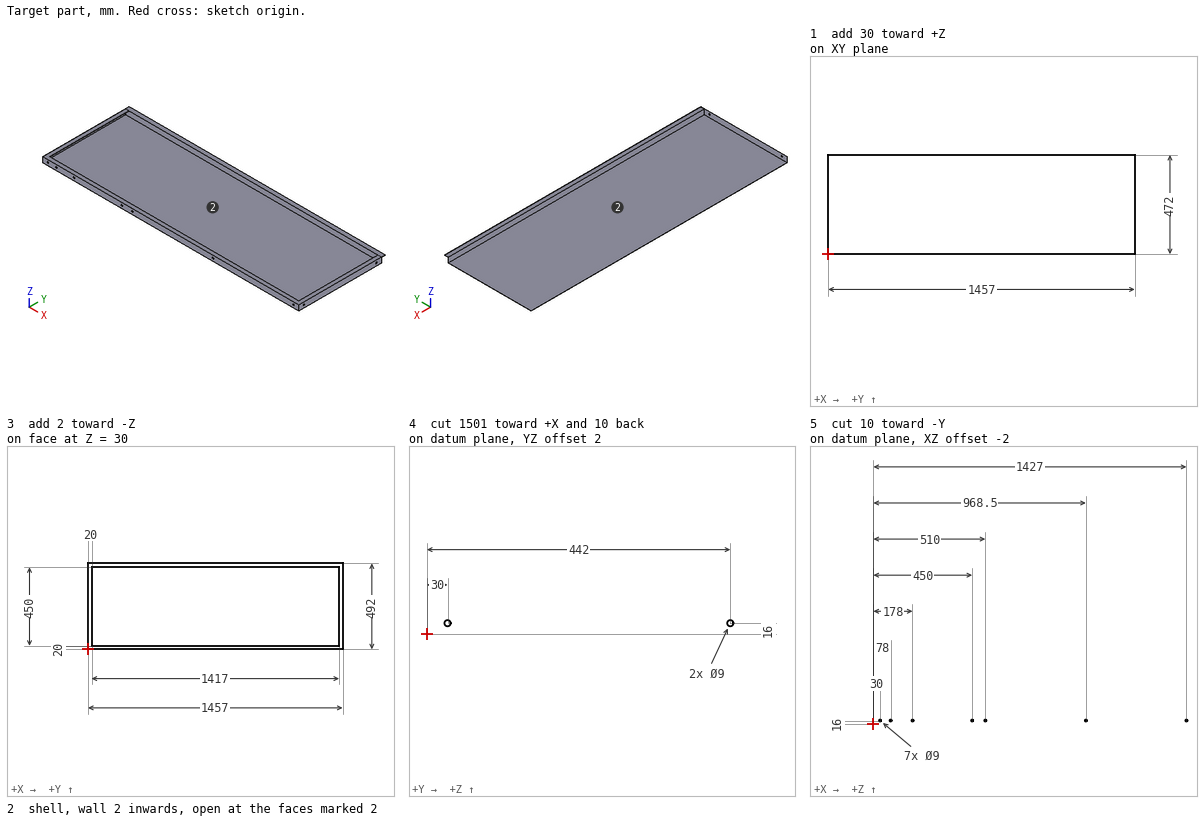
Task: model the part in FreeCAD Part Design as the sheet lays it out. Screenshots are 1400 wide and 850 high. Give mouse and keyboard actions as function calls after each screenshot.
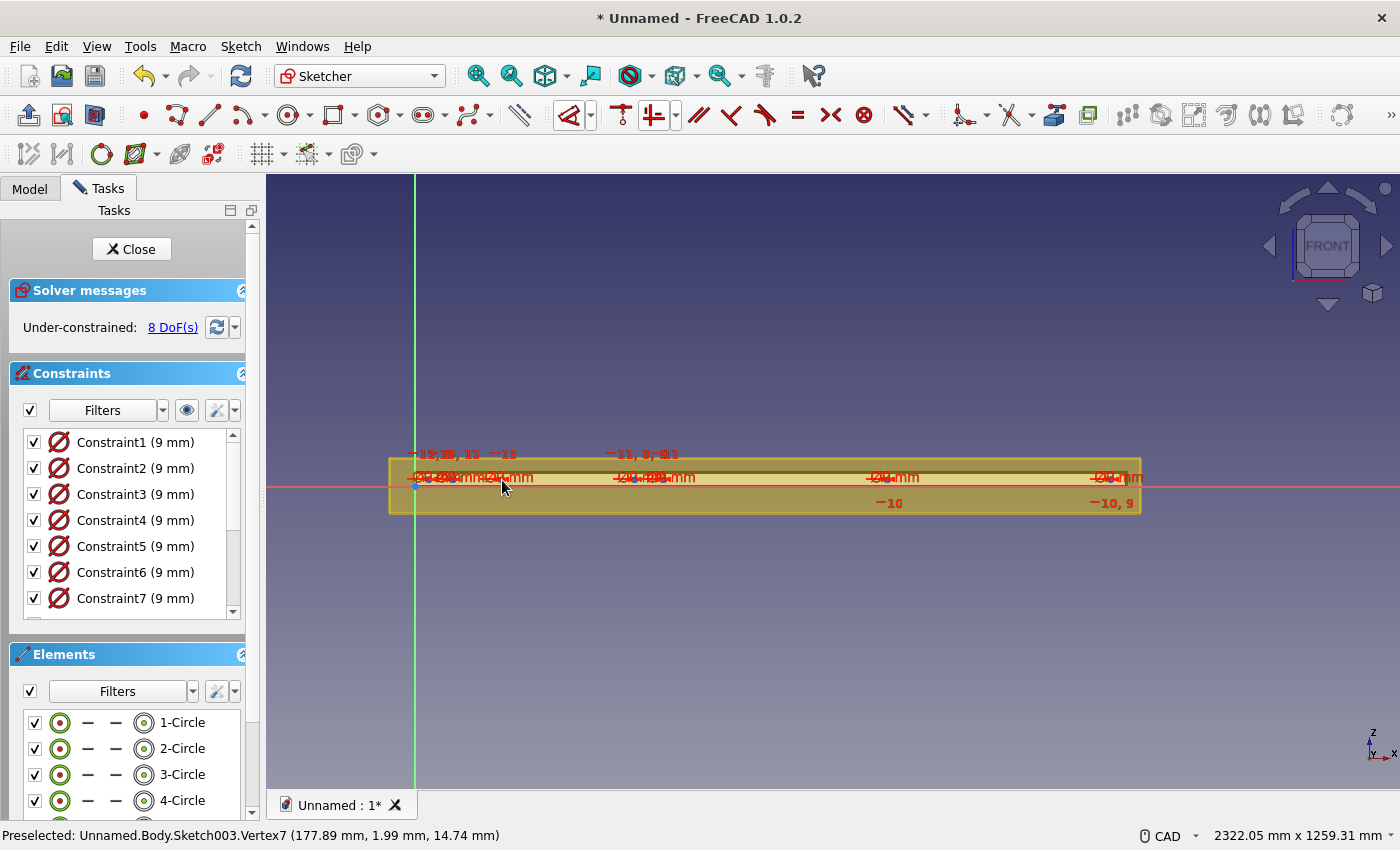
scroll(430, 479, up, 5)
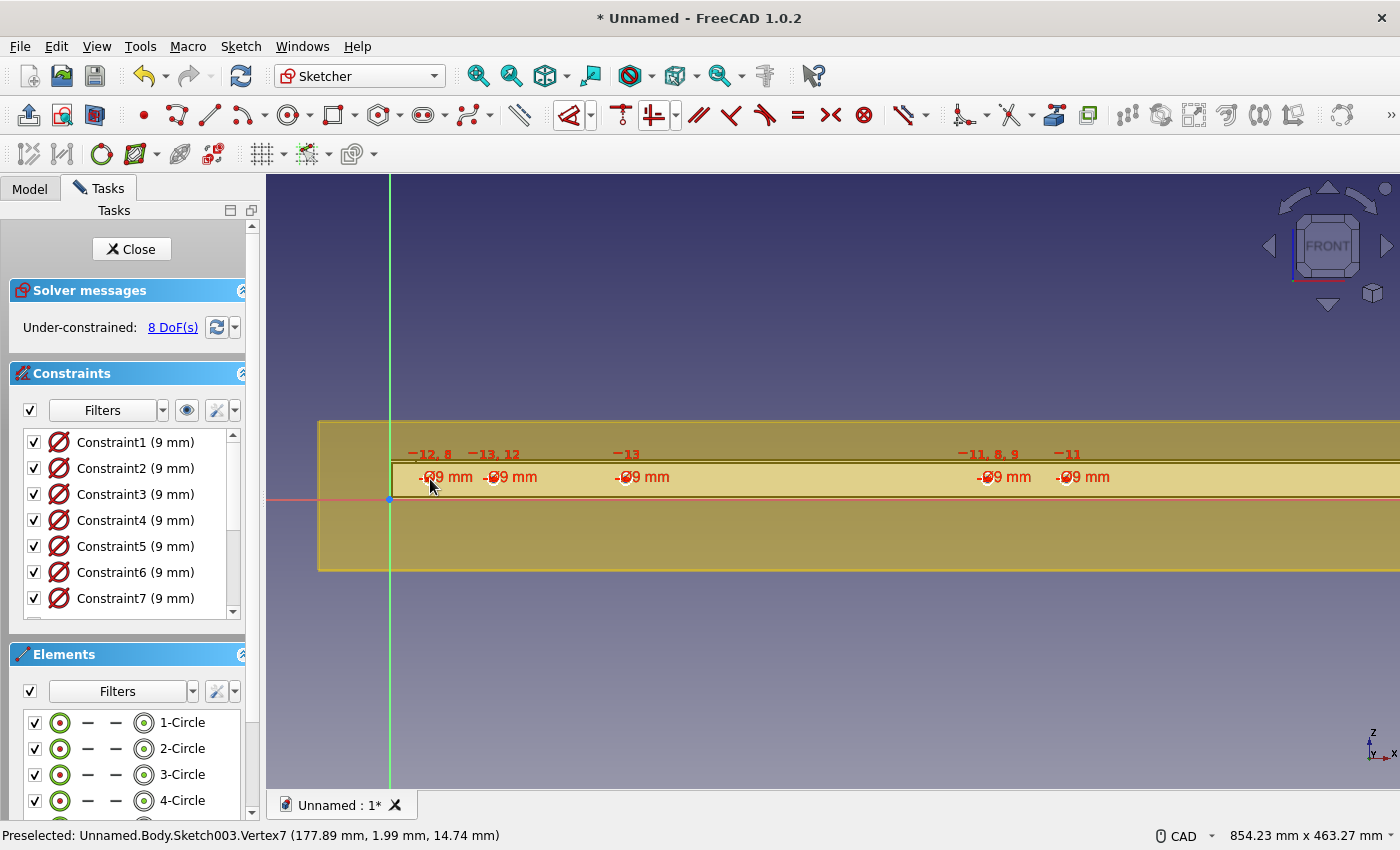
click(429, 479)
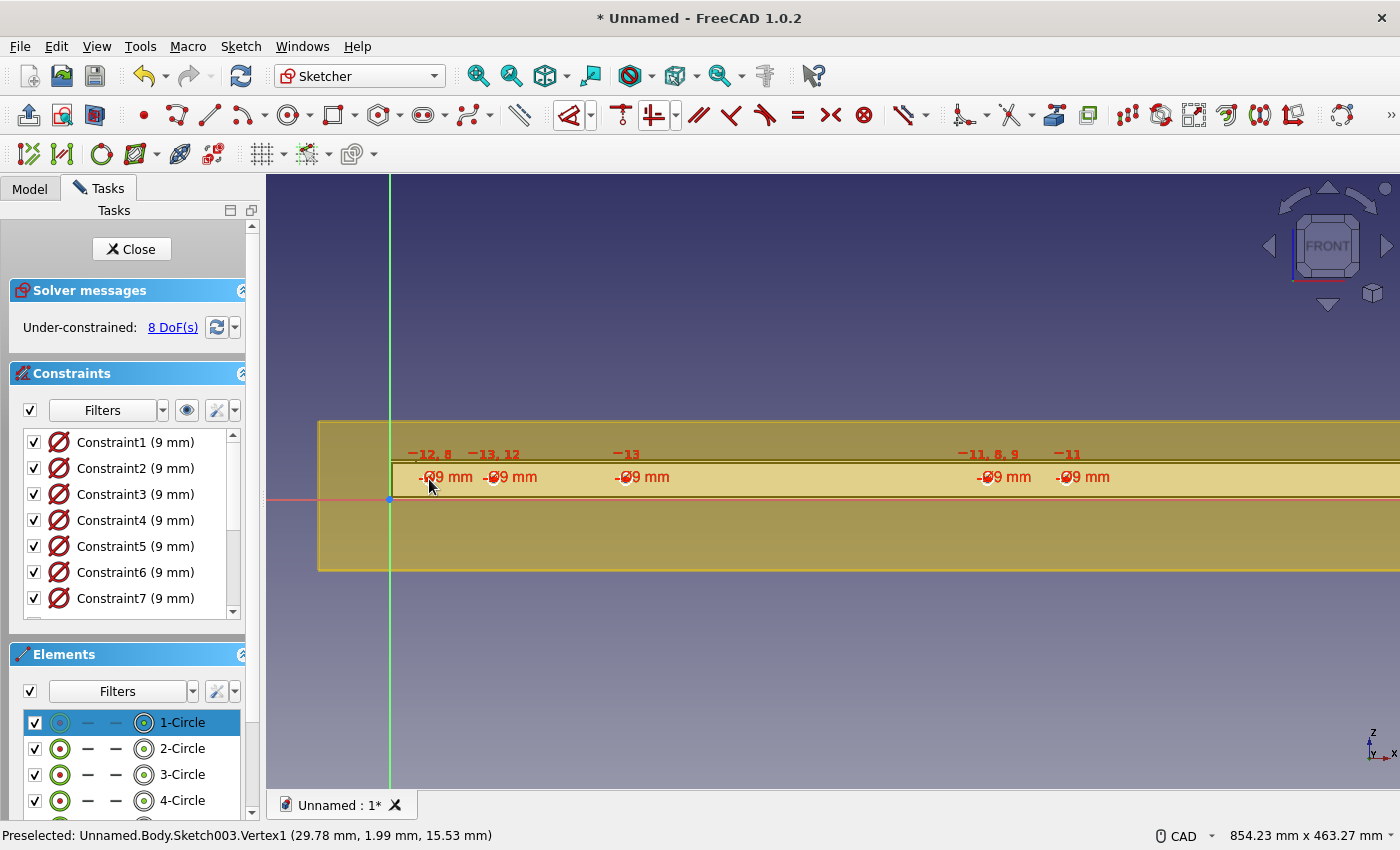
key(l)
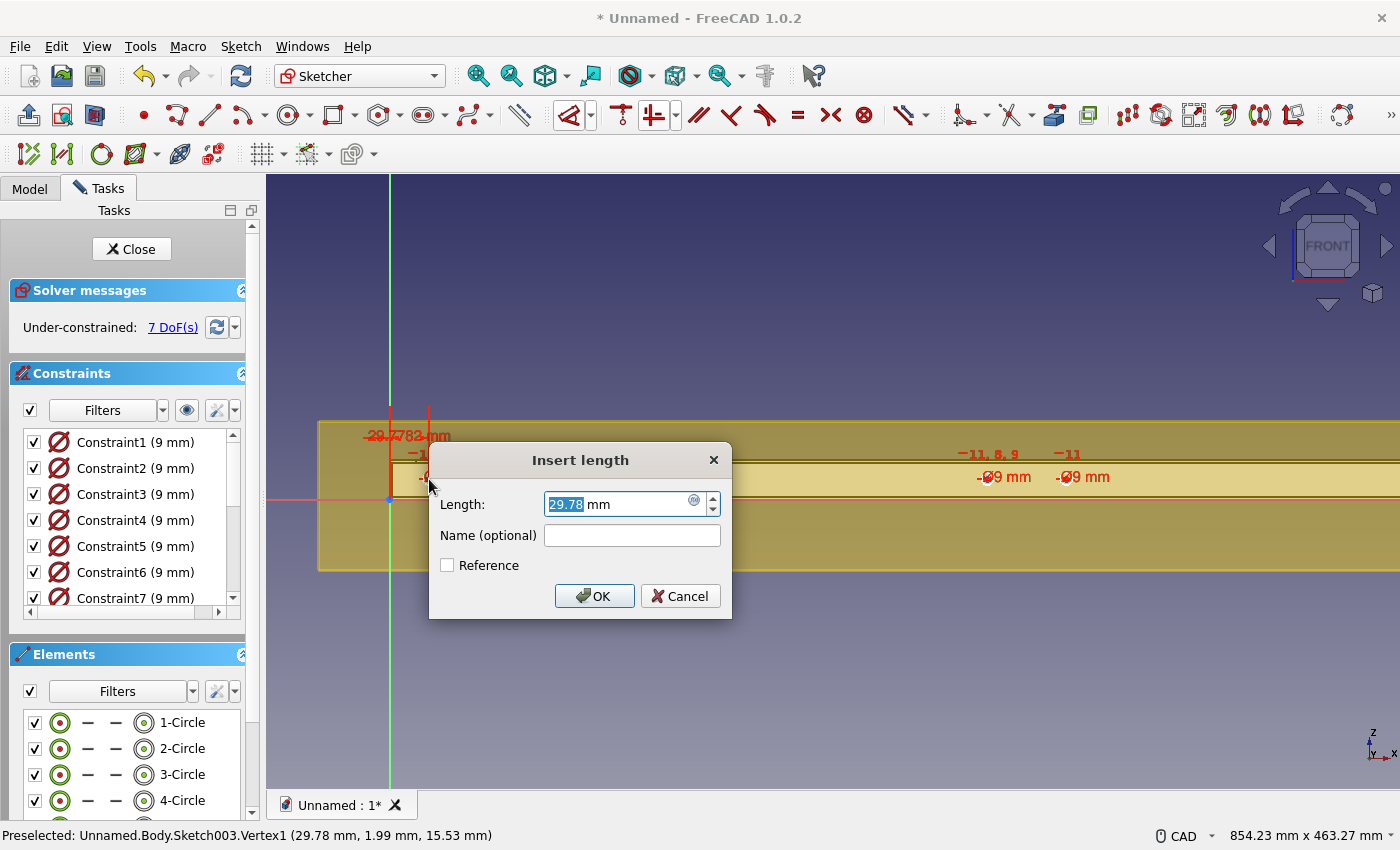
text(30)
key(Return)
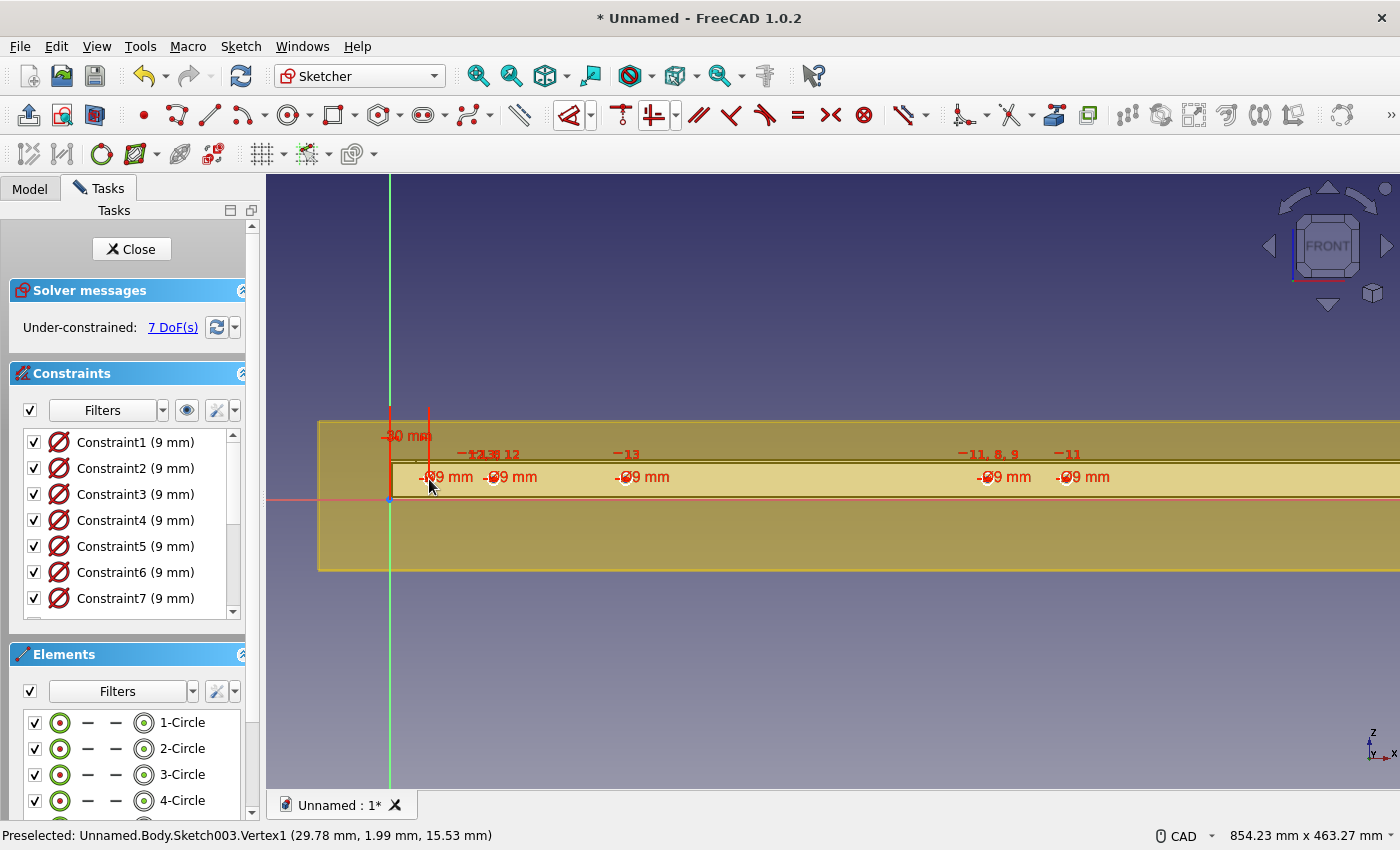
scroll(429, 479, up, 4)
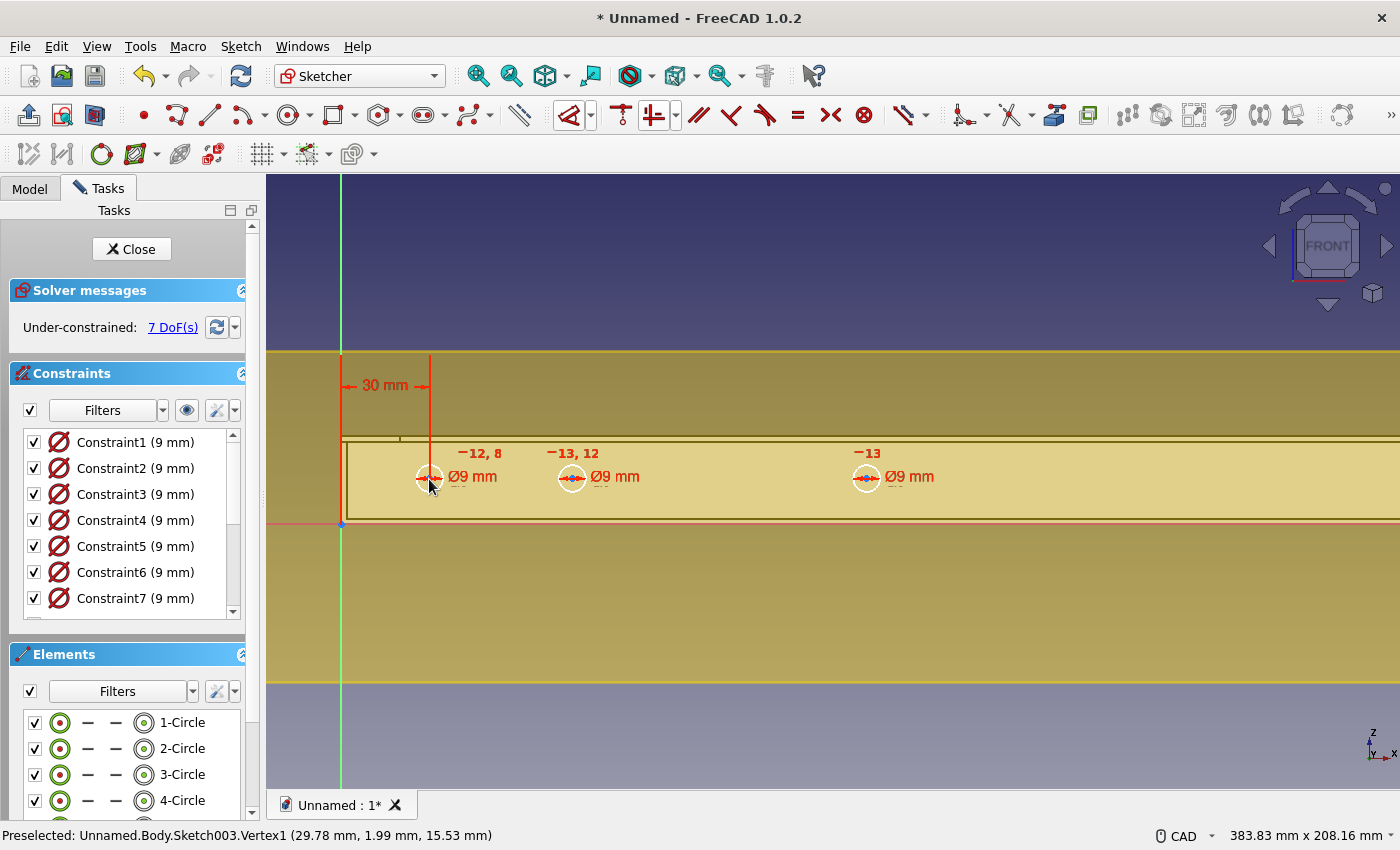
click(430, 479)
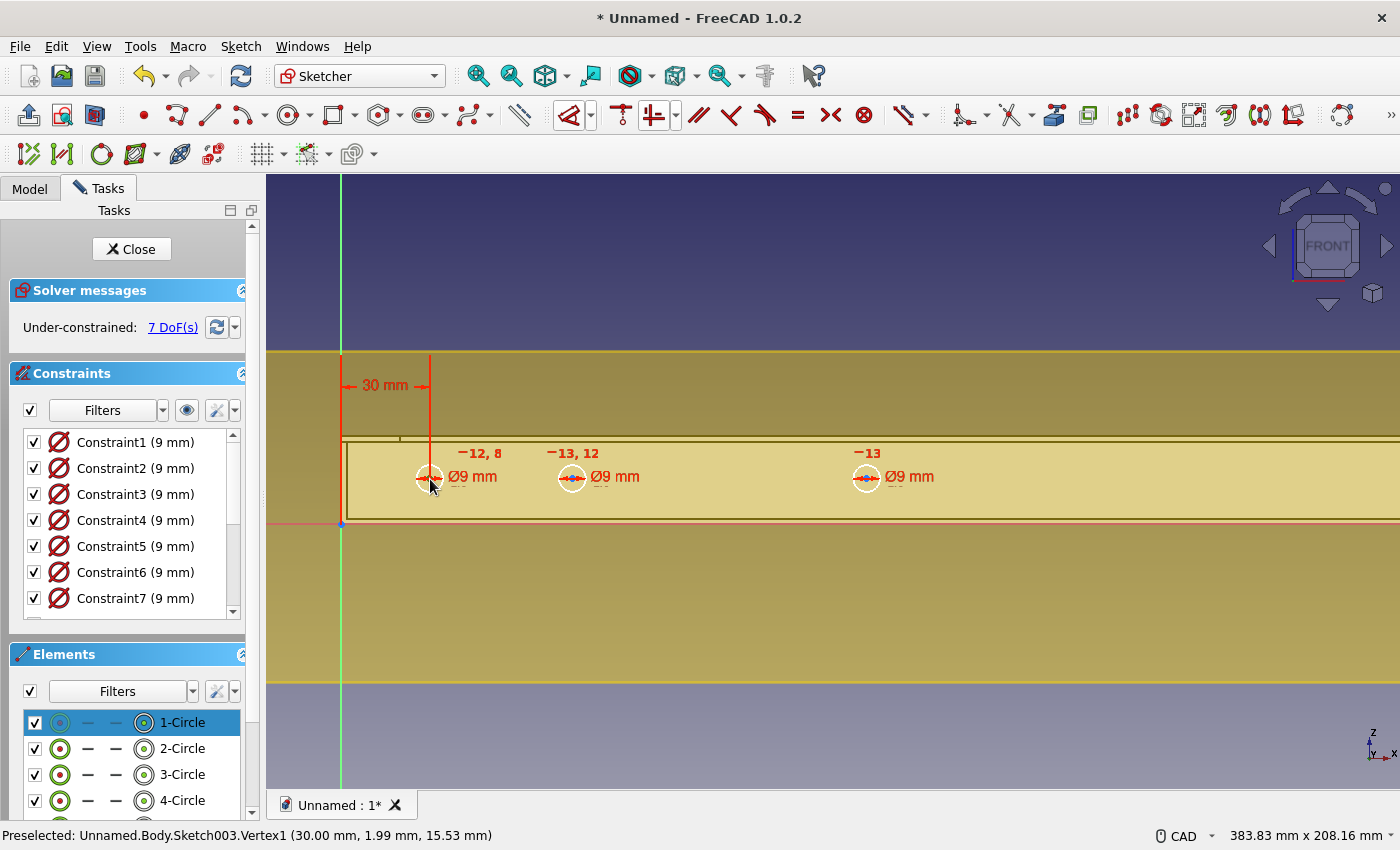
key(i)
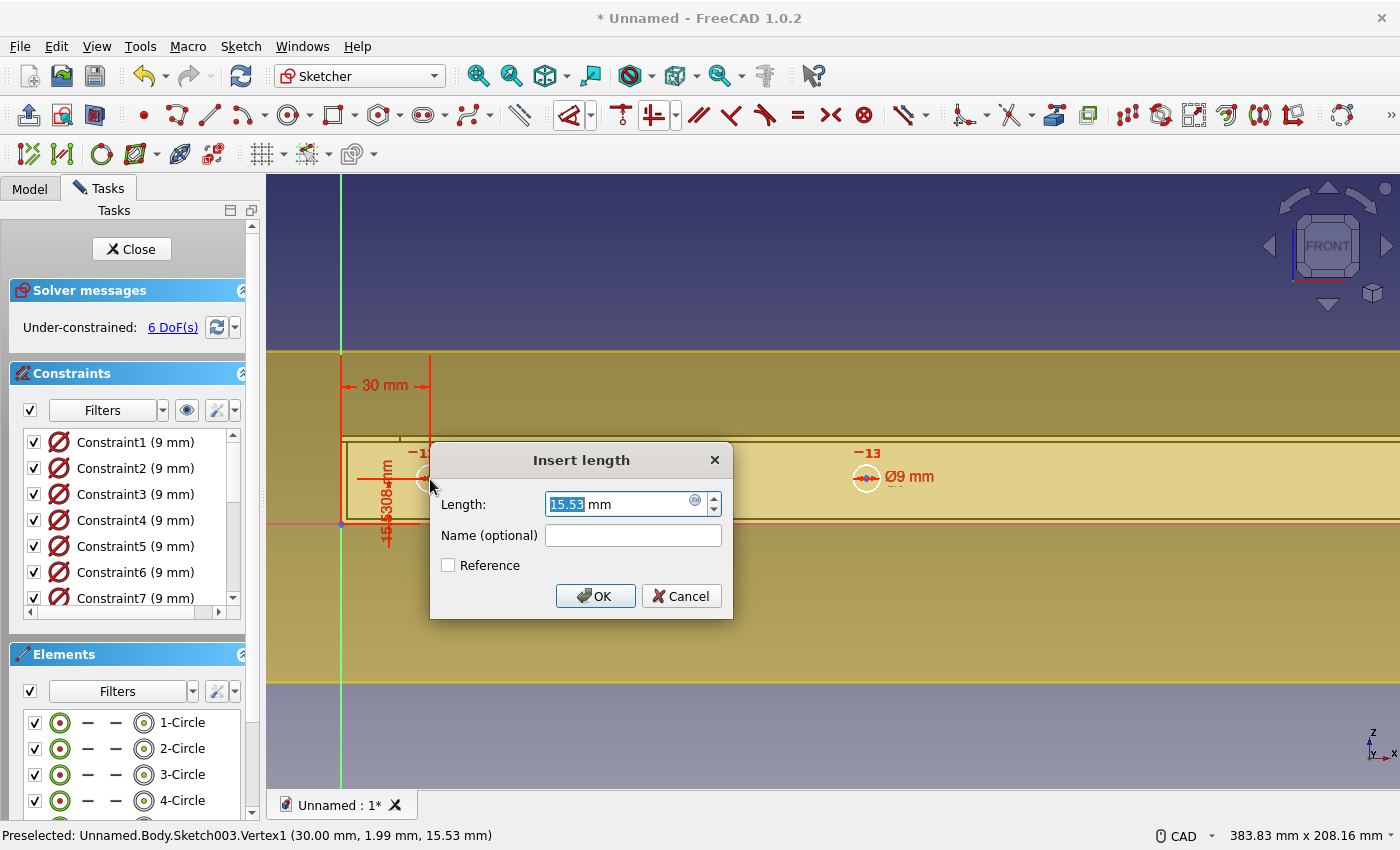
text(16)
key(Return)